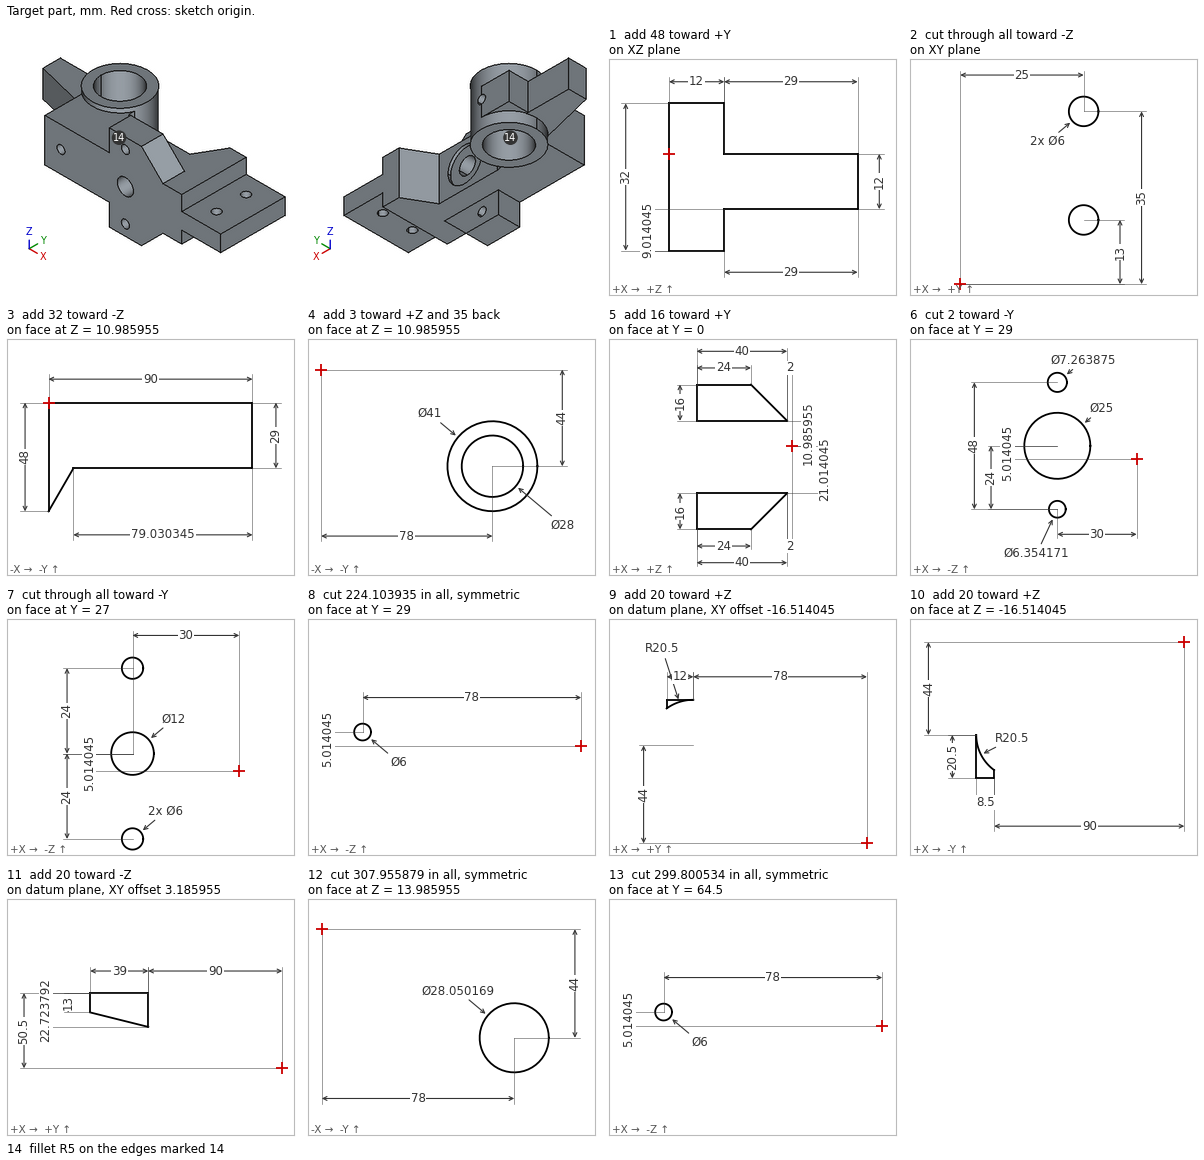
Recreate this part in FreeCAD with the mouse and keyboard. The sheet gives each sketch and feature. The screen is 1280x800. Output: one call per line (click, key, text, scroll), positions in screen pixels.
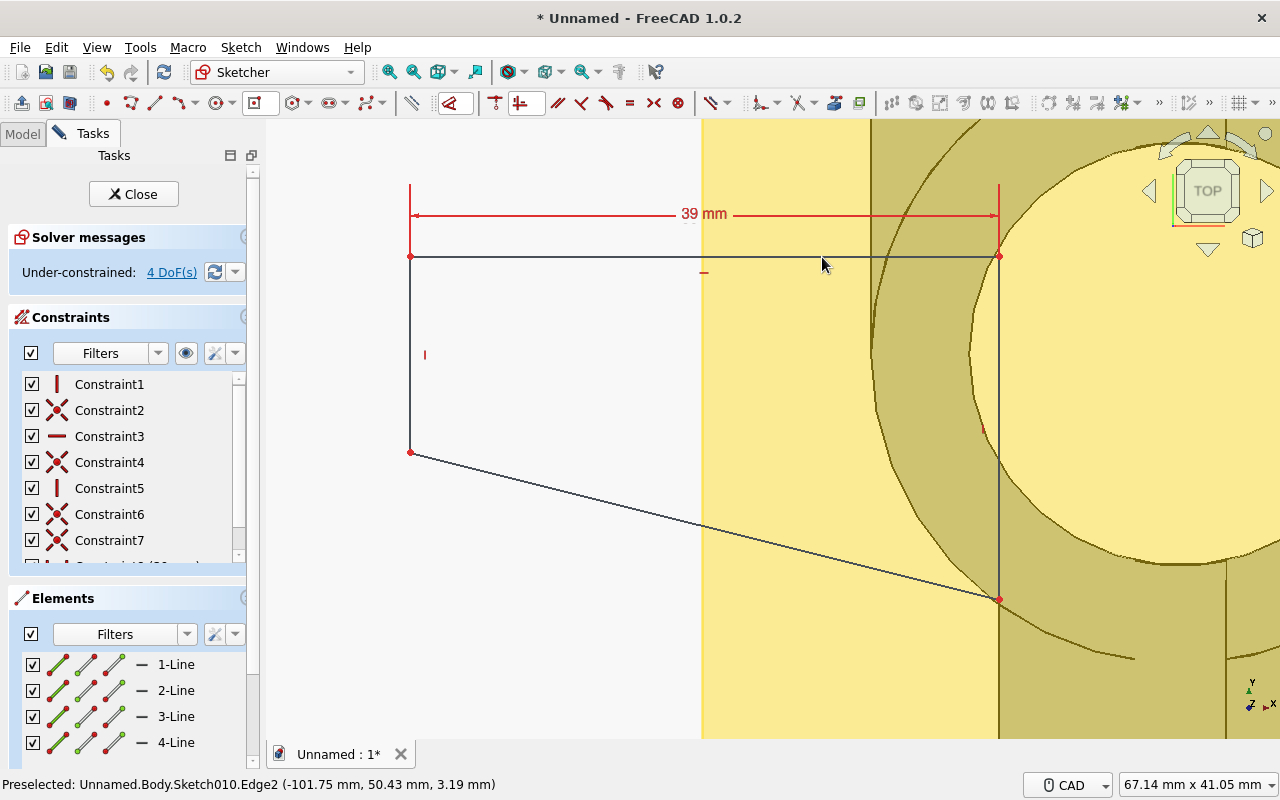
click(410, 316)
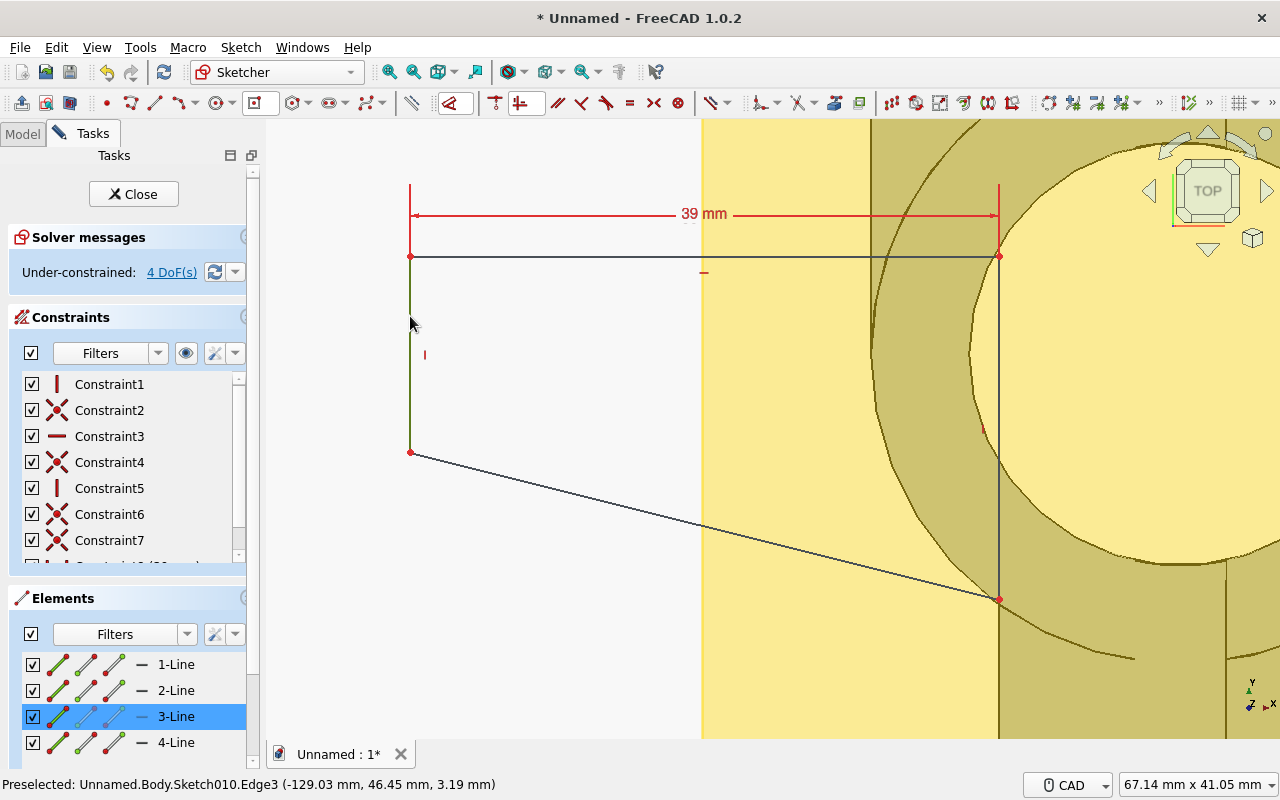
key(i)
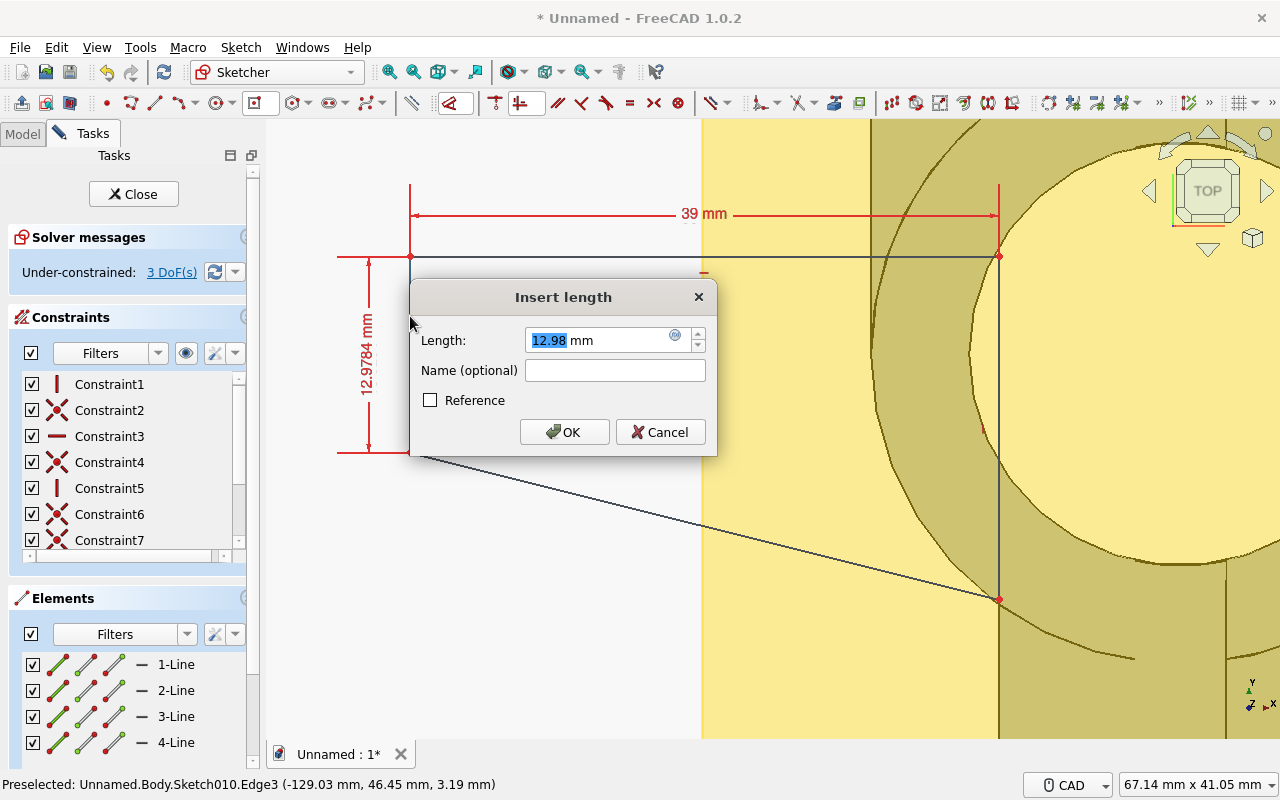
text(13)
key(Return)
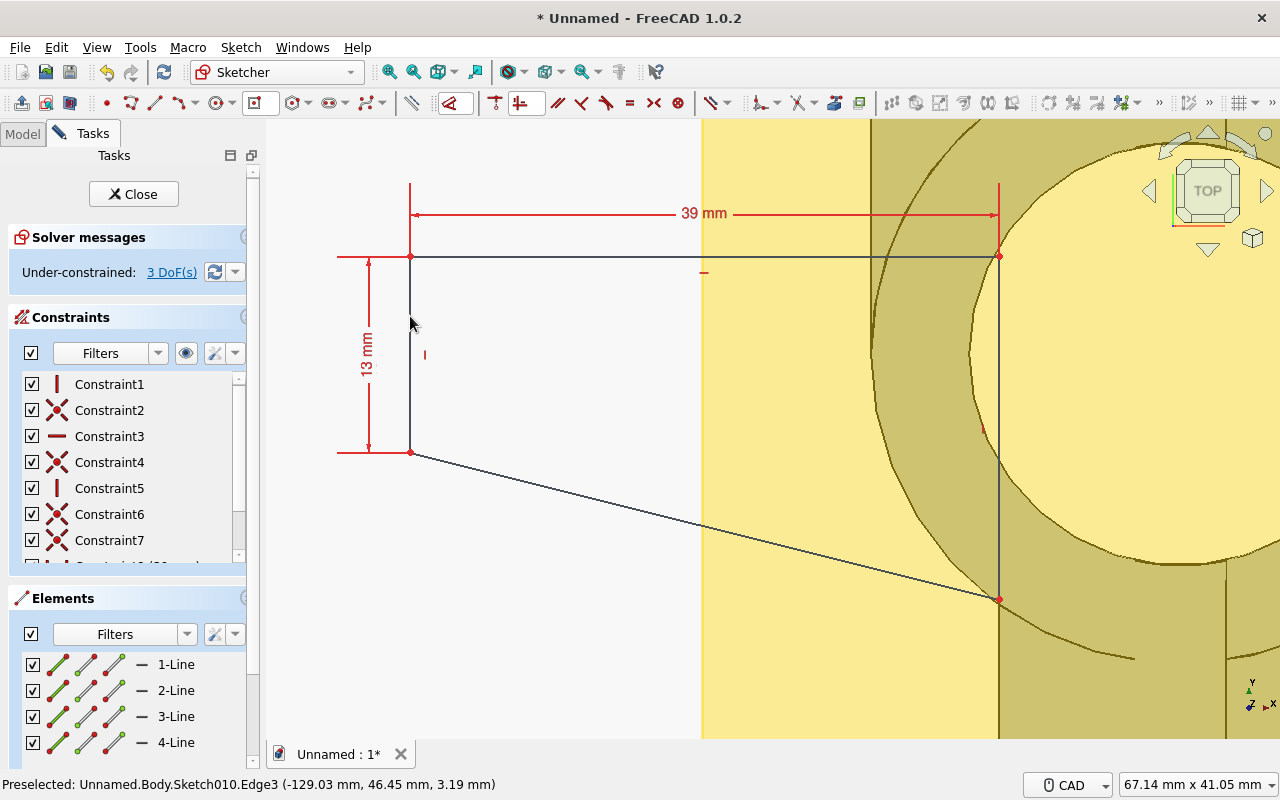
click(999, 600)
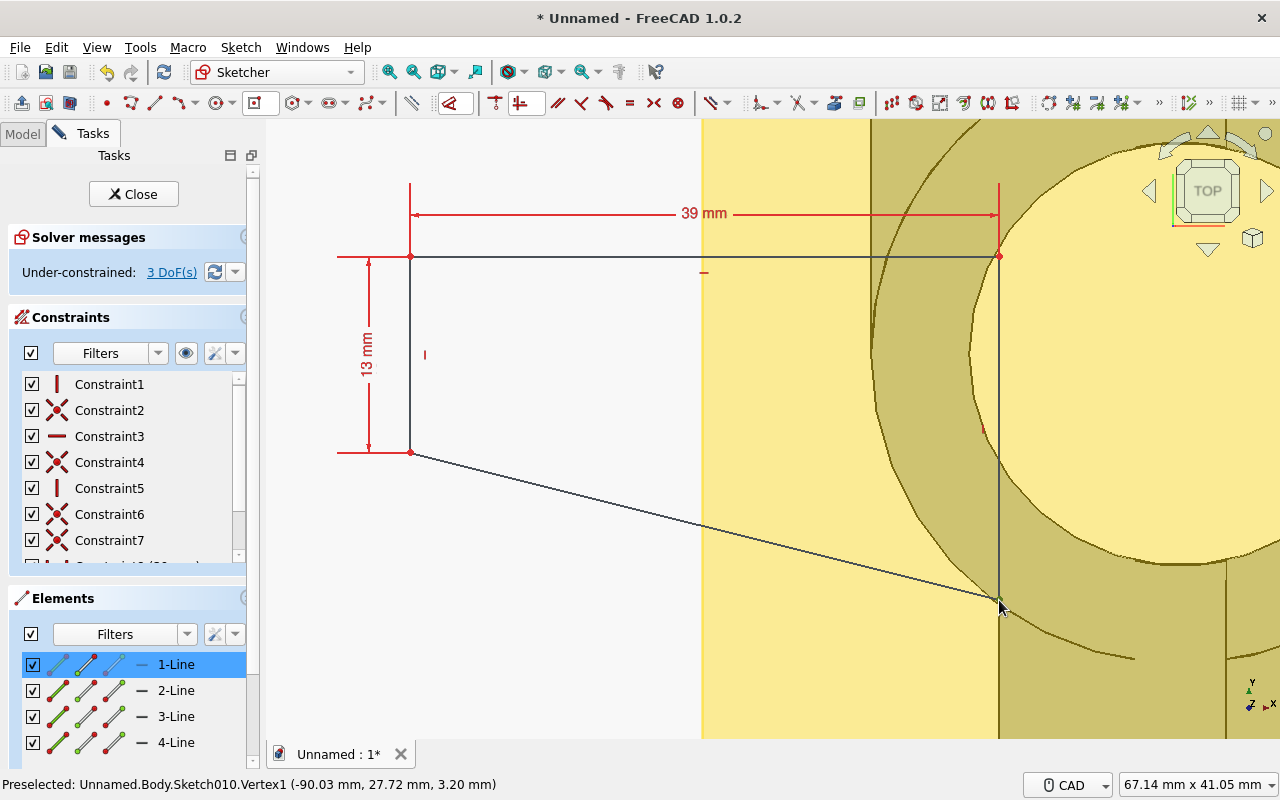
key(l)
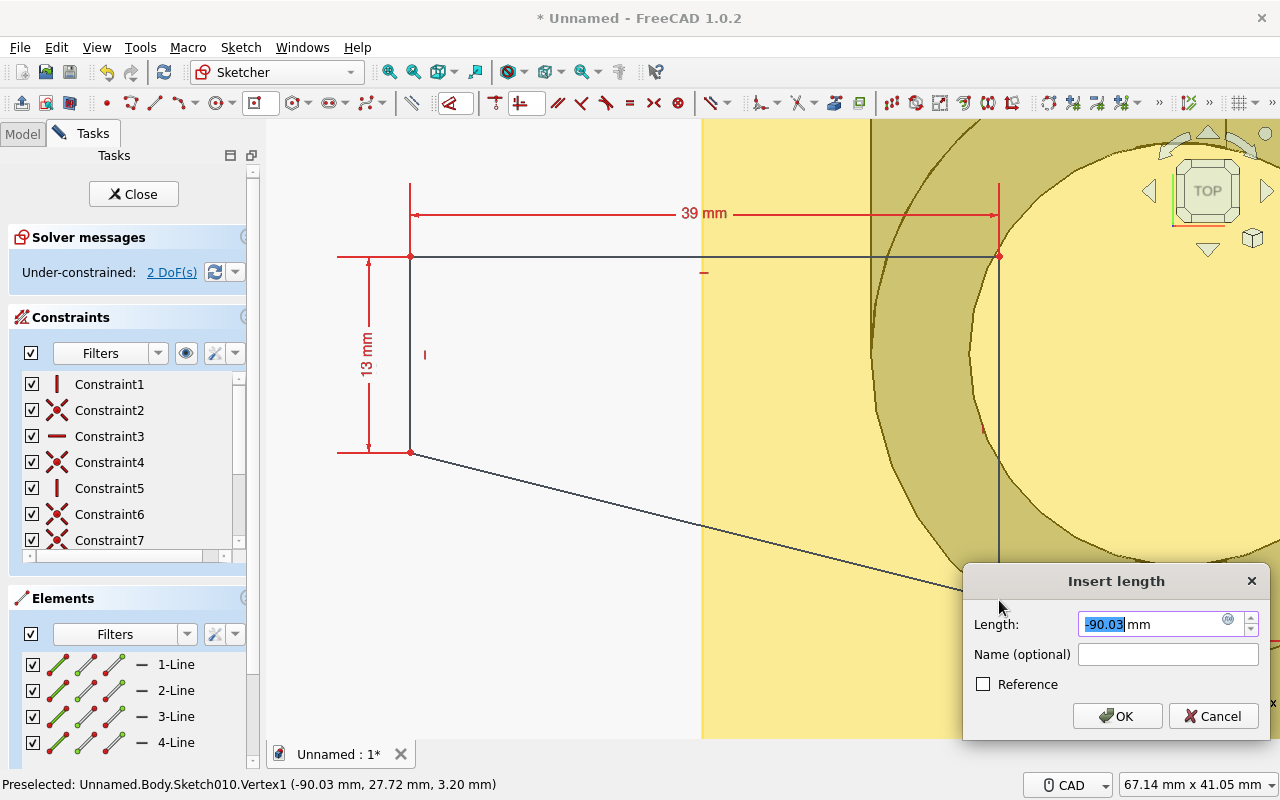
text(-90)
key(Return)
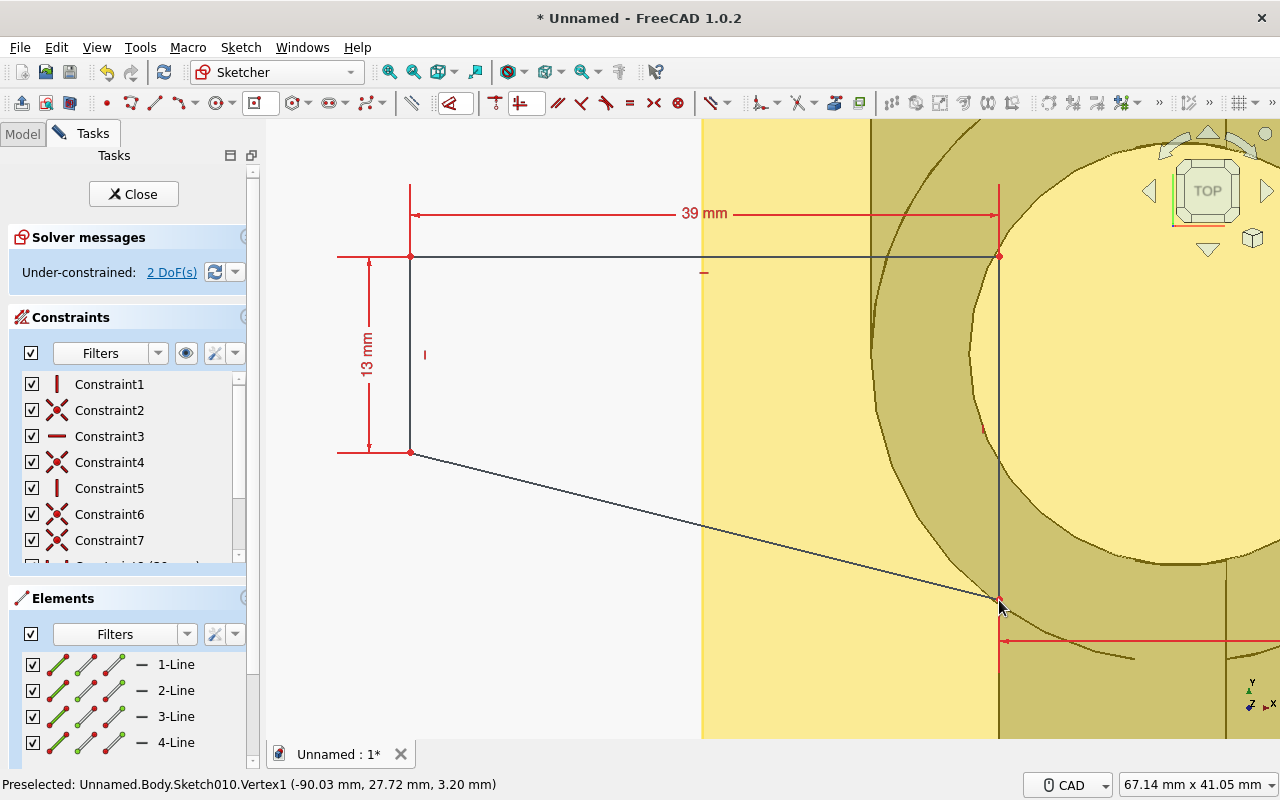
click(999, 257)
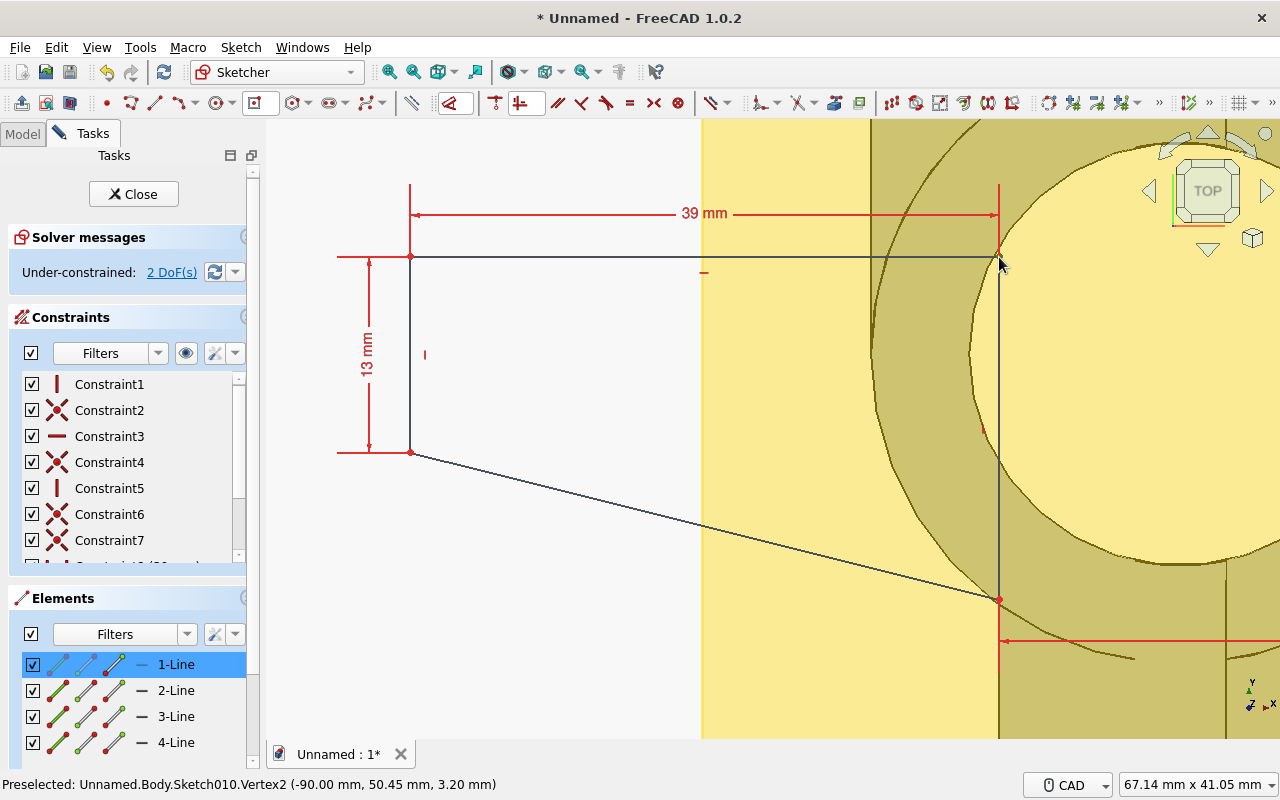
click(468, 104)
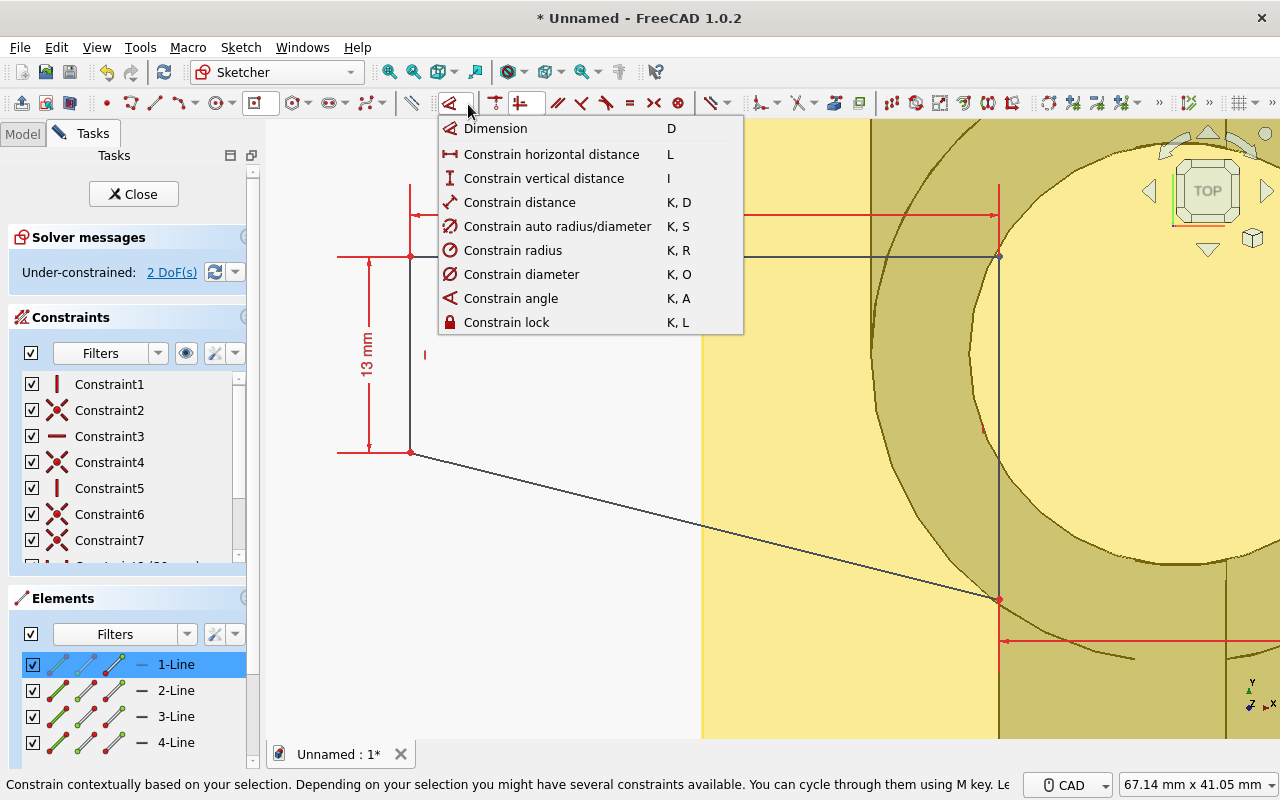
click(591, 178)